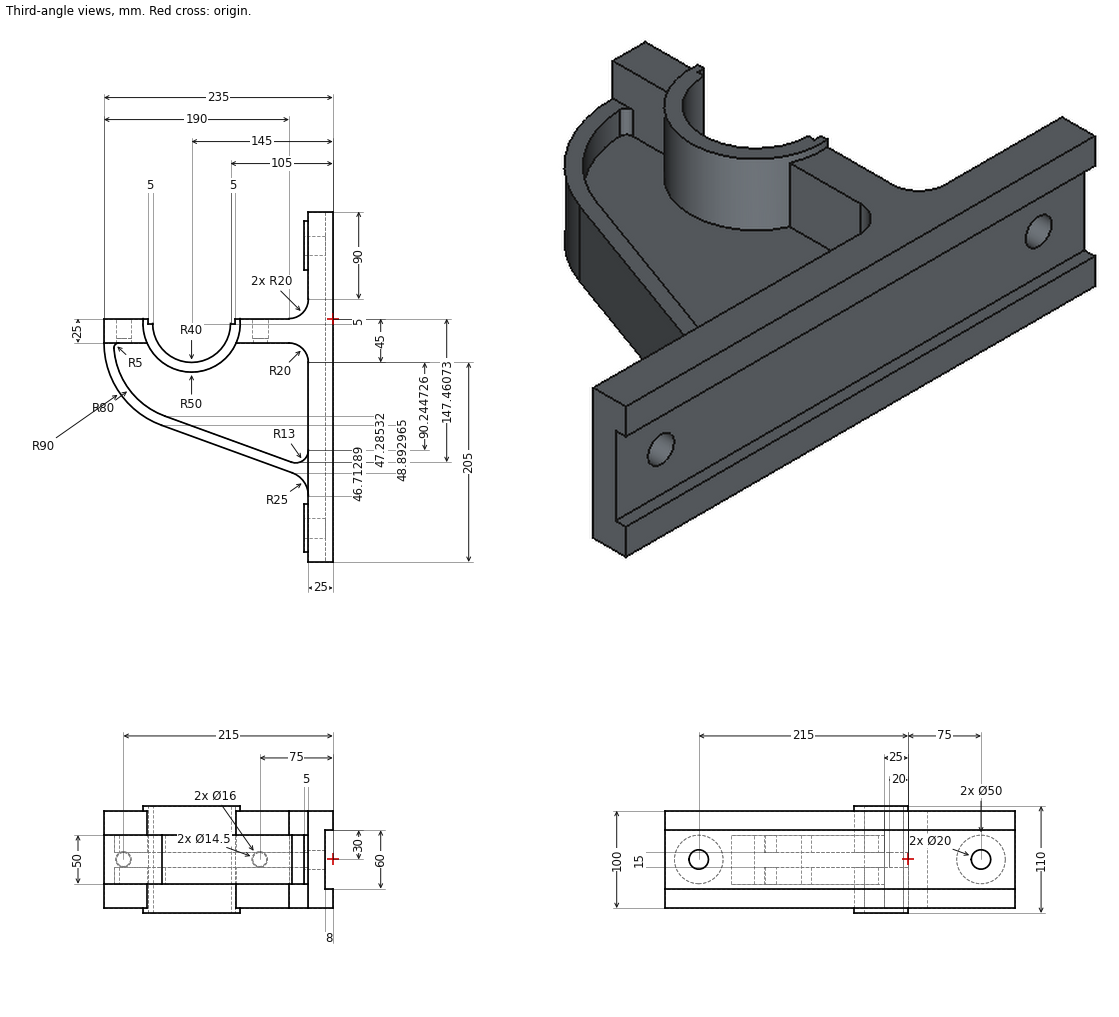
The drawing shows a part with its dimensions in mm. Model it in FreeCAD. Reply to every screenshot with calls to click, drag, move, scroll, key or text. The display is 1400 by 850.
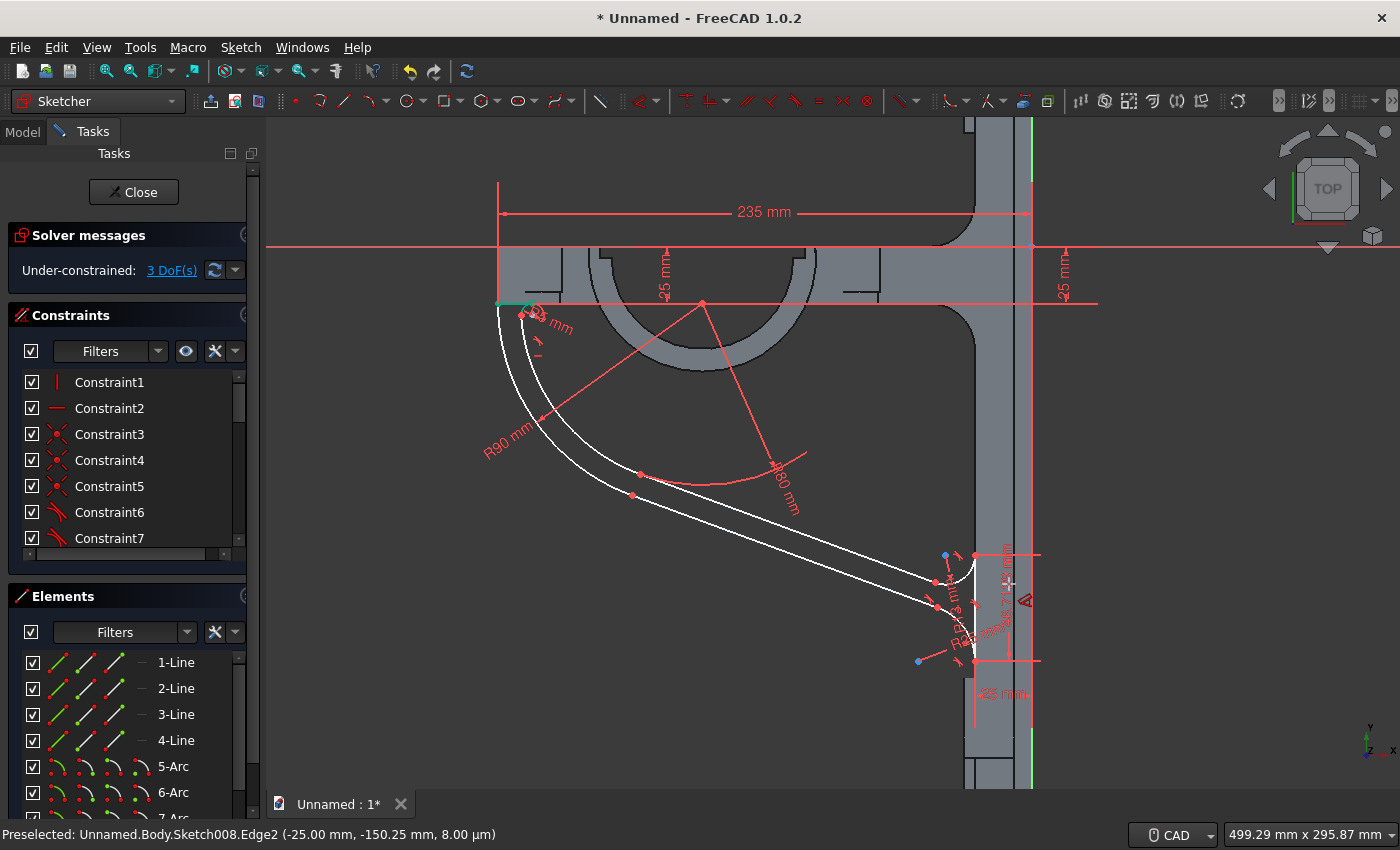
click(847, 550)
click(969, 529)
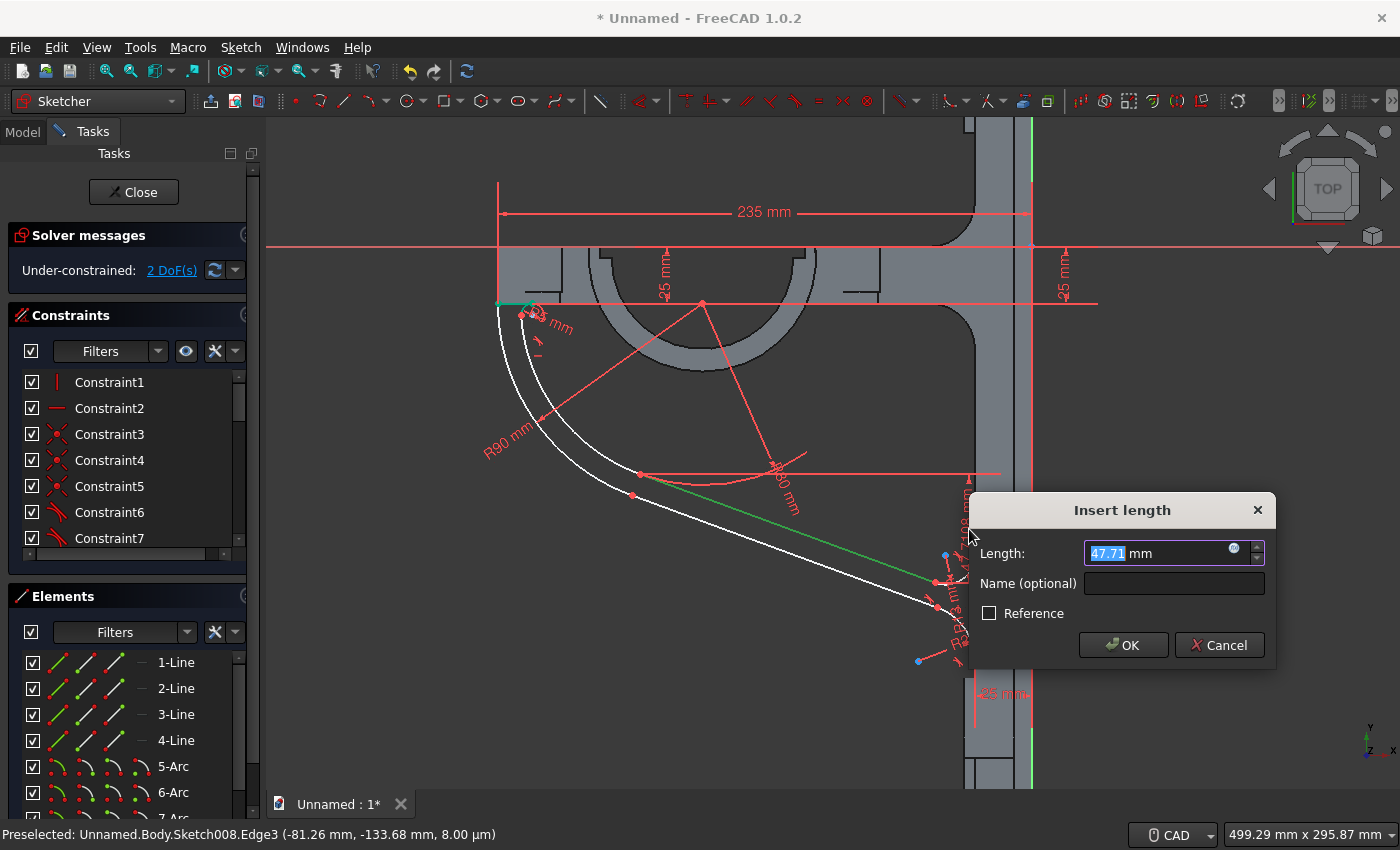
text(47.28532)
key(Return)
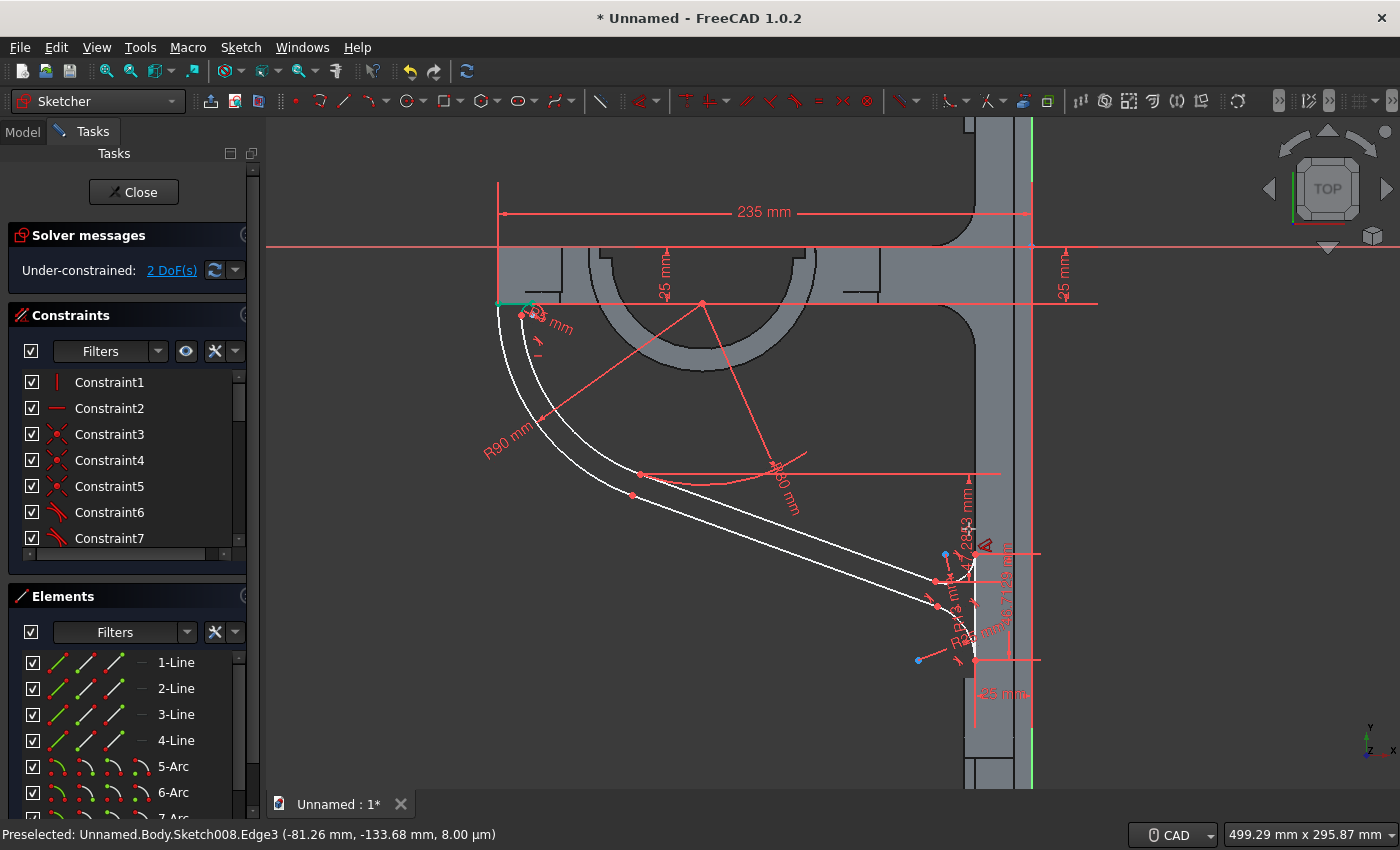
click(935, 582)
click(1066, 414)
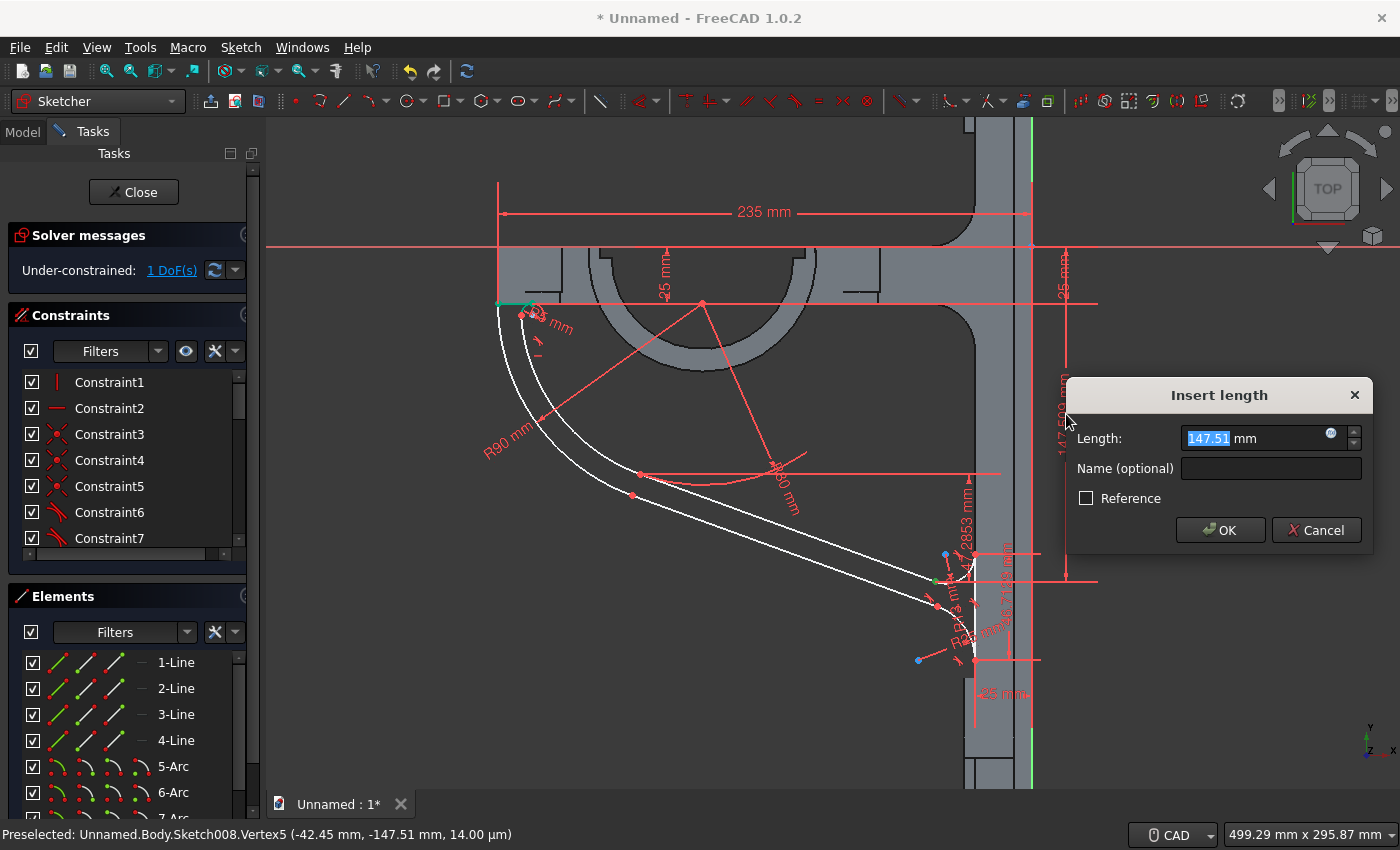
text(147.46073)
key(Return)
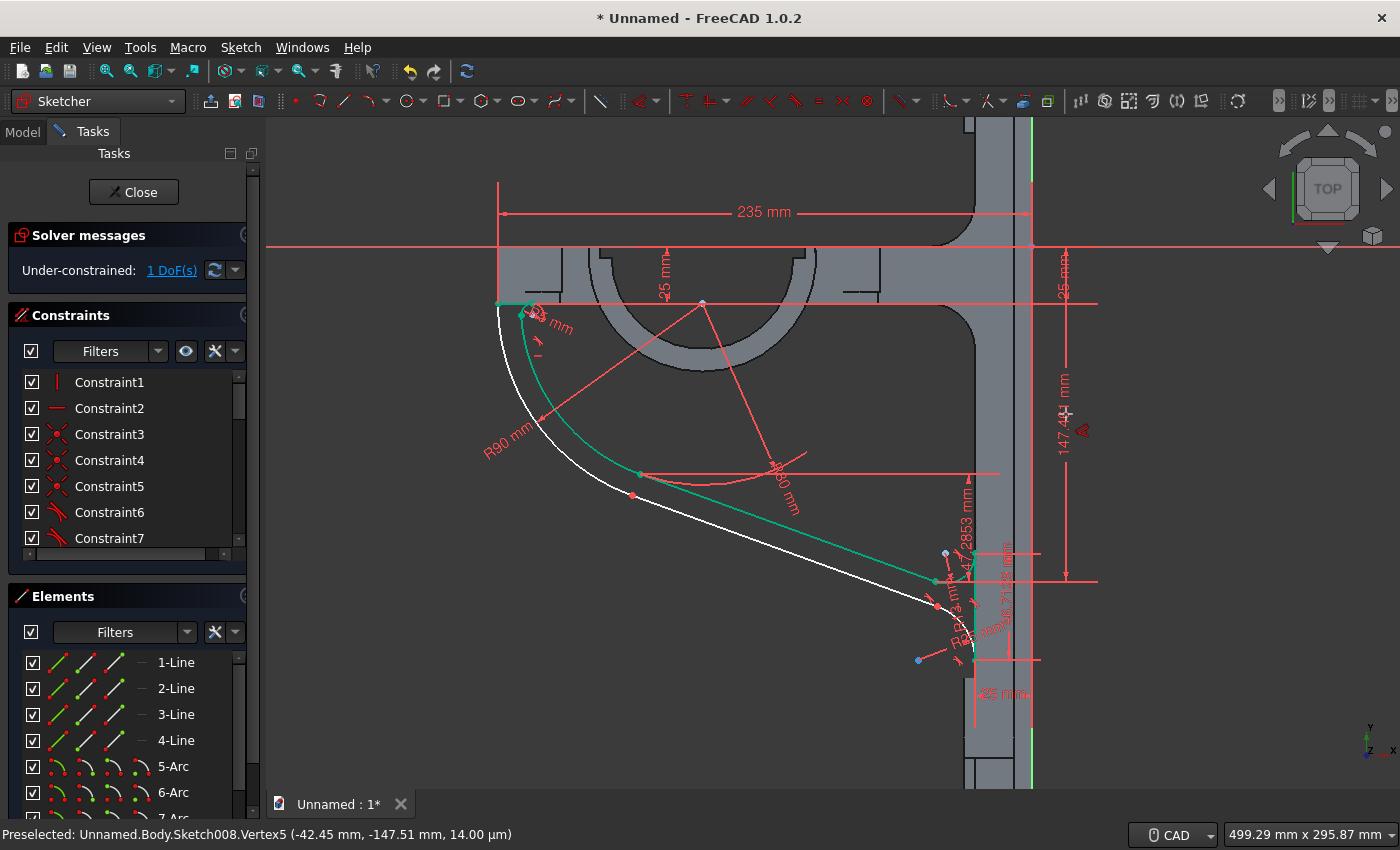
click(724, 529)
click(599, 551)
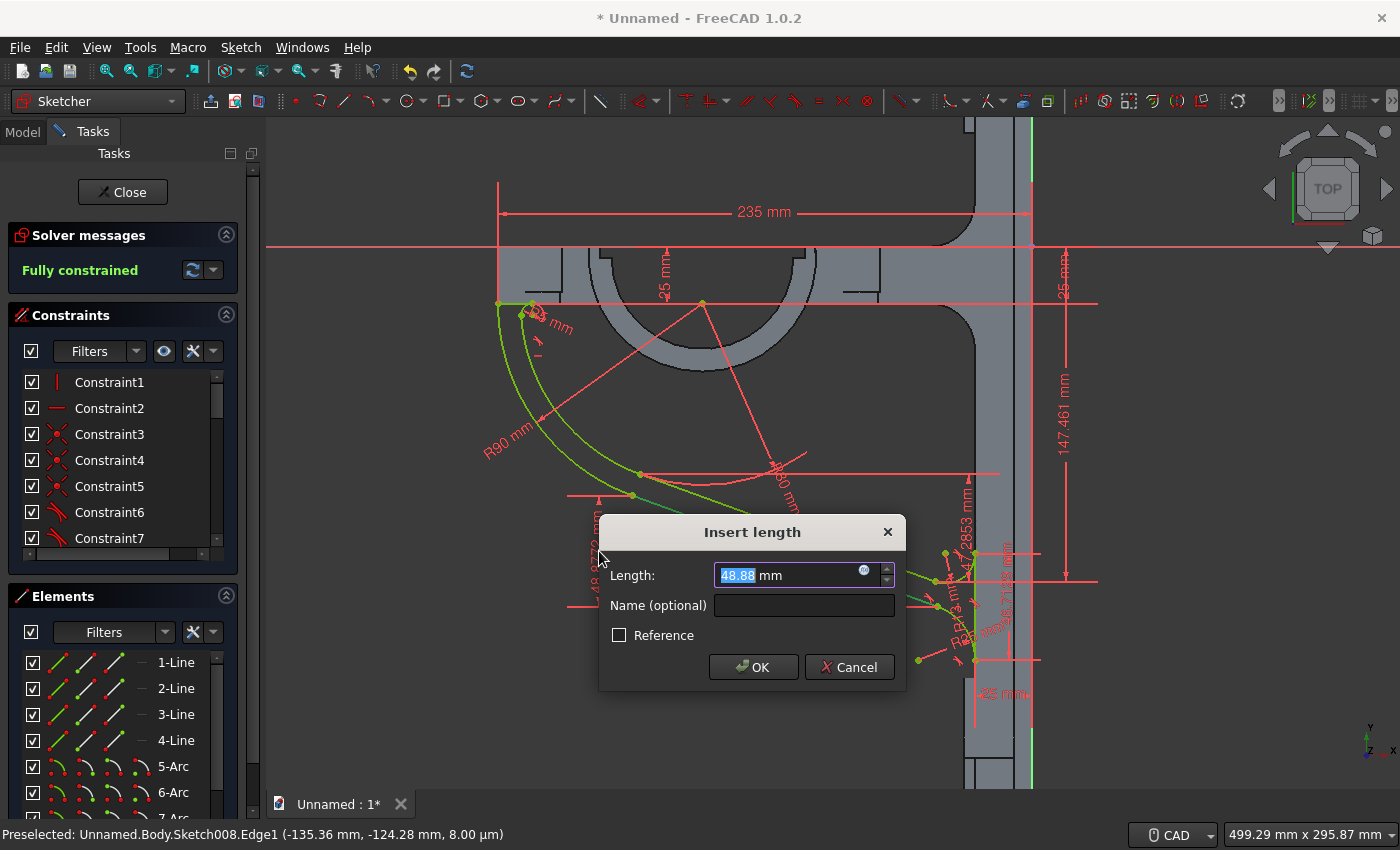
text(48.892965)
key(Return)
key(Escape)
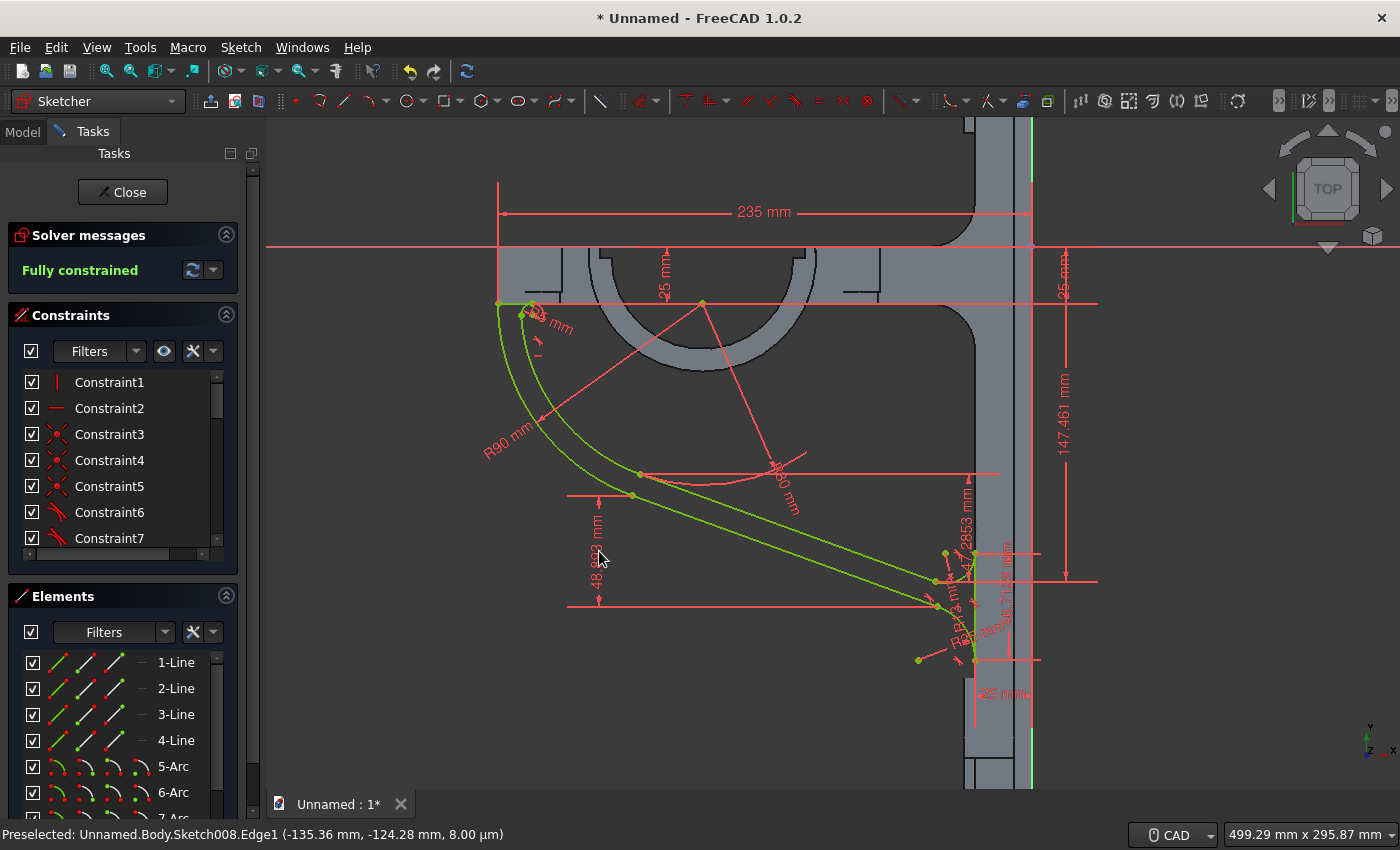
click(123, 192)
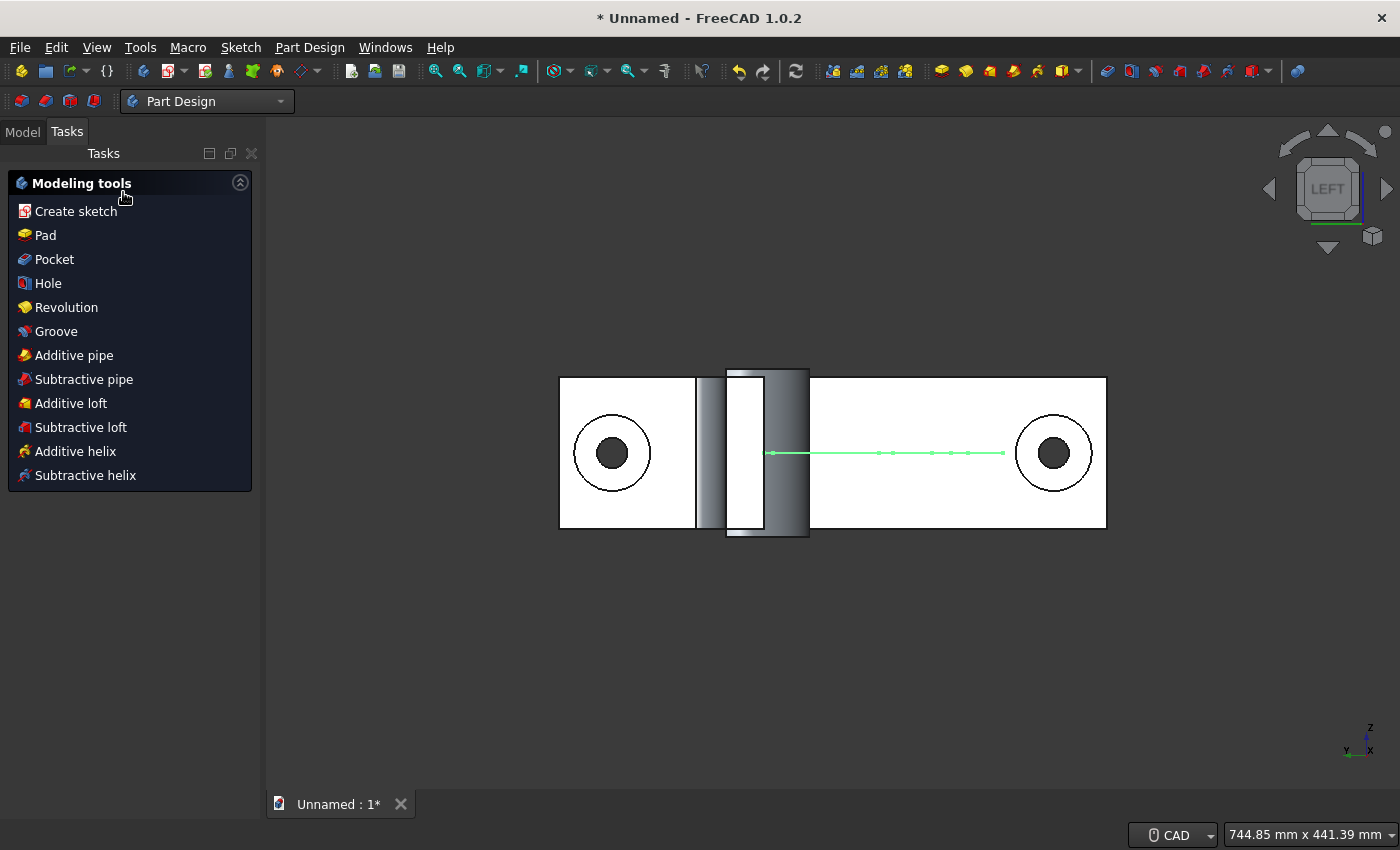
click(942, 72)